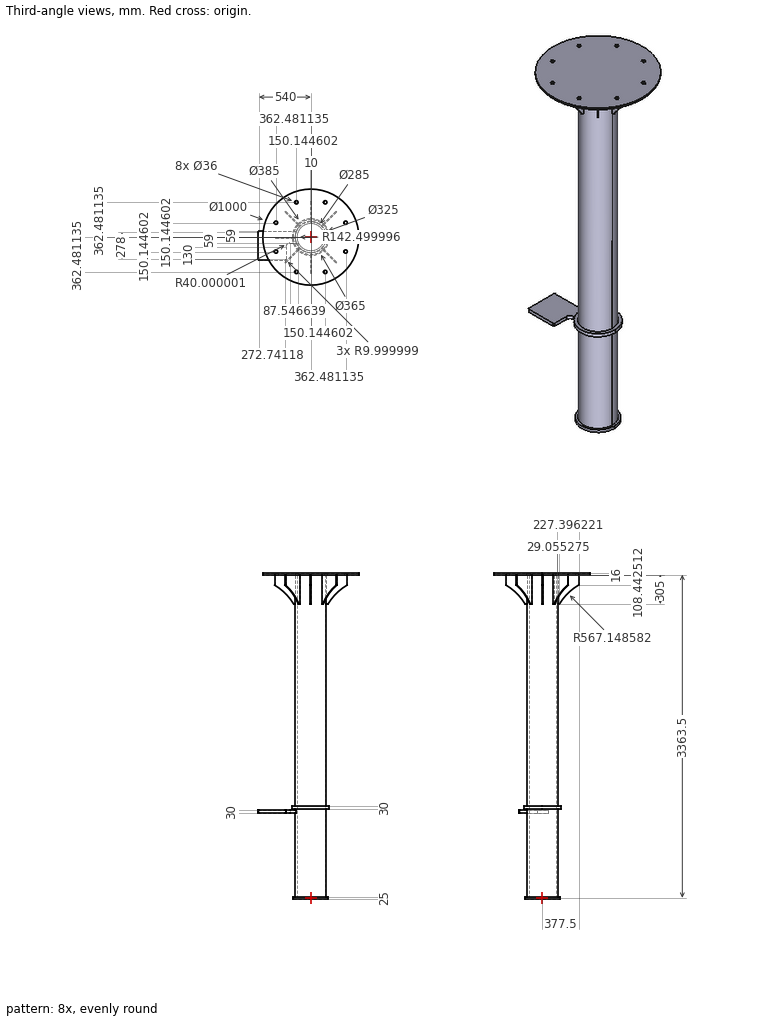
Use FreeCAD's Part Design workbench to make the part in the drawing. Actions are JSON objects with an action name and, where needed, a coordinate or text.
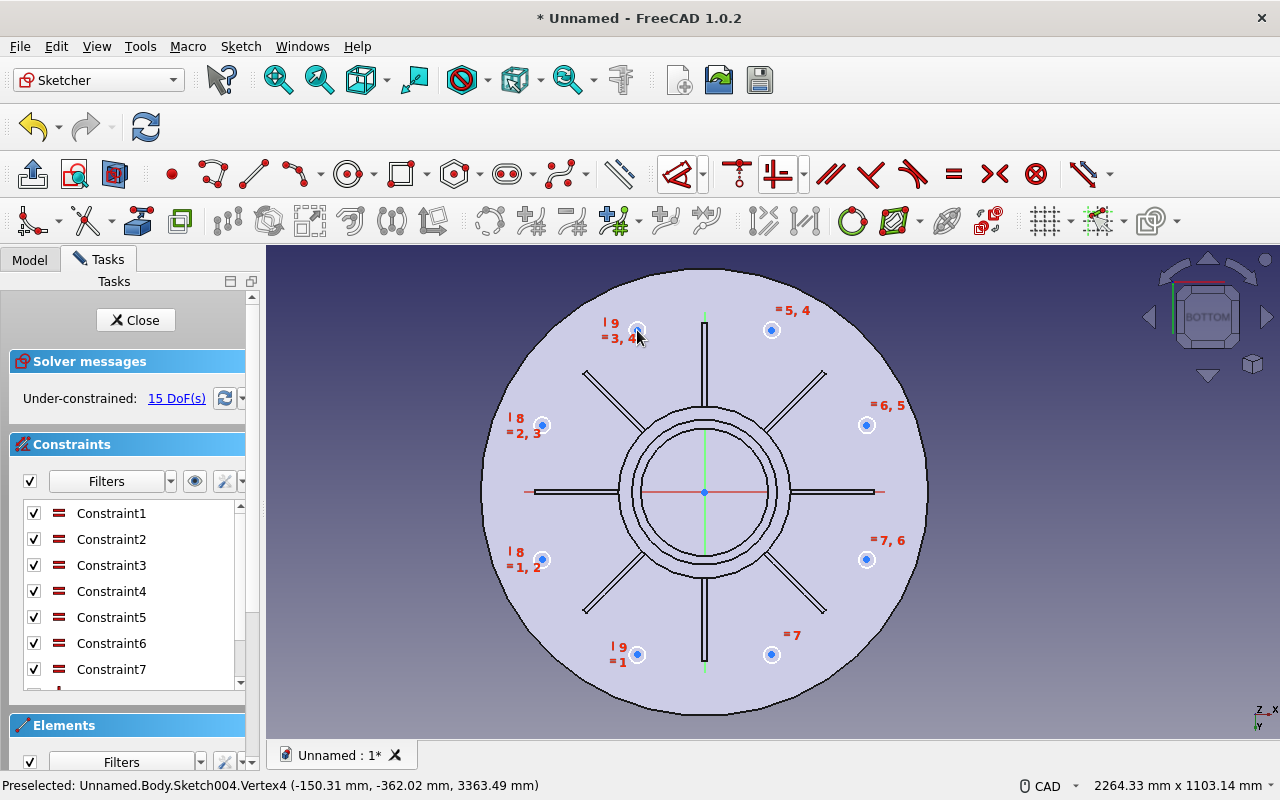
{"action": "left_click", "coordinate": [637, 330]}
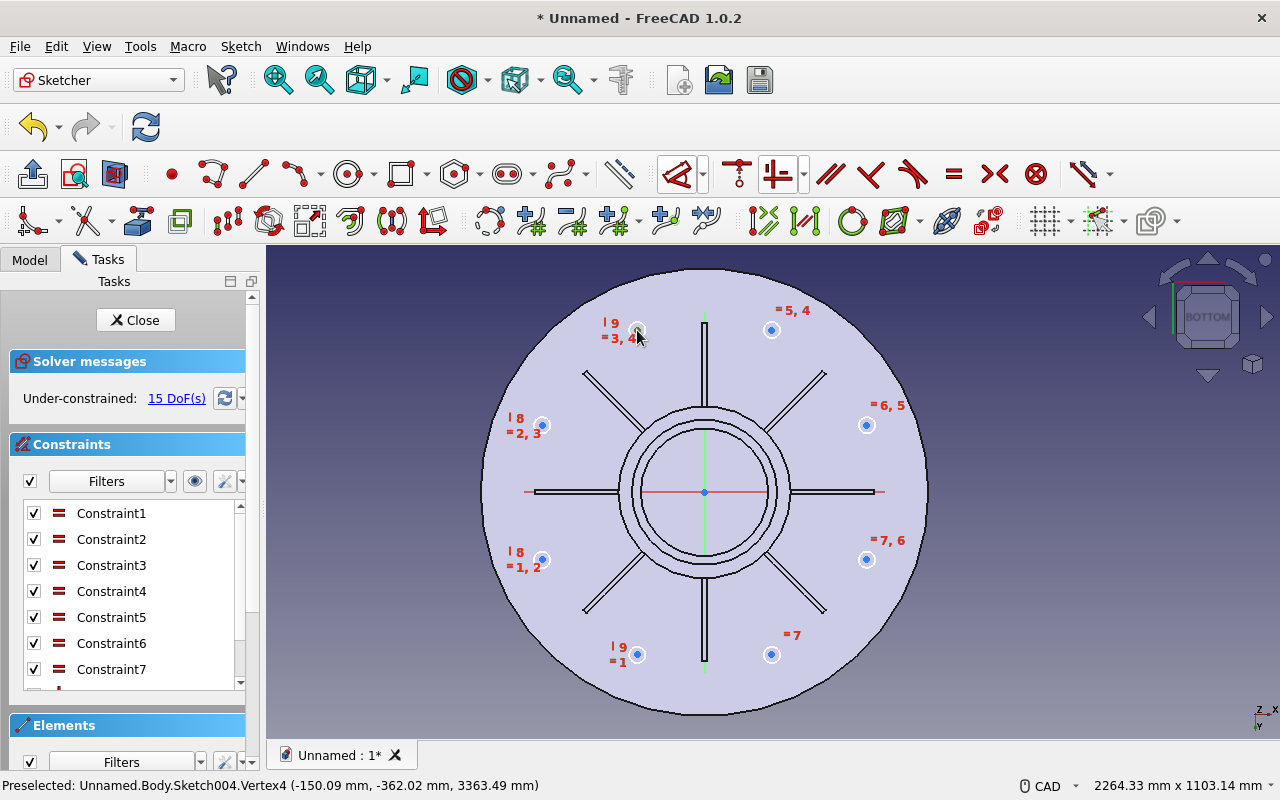
{"action": "left_click", "coordinate": [772, 330]}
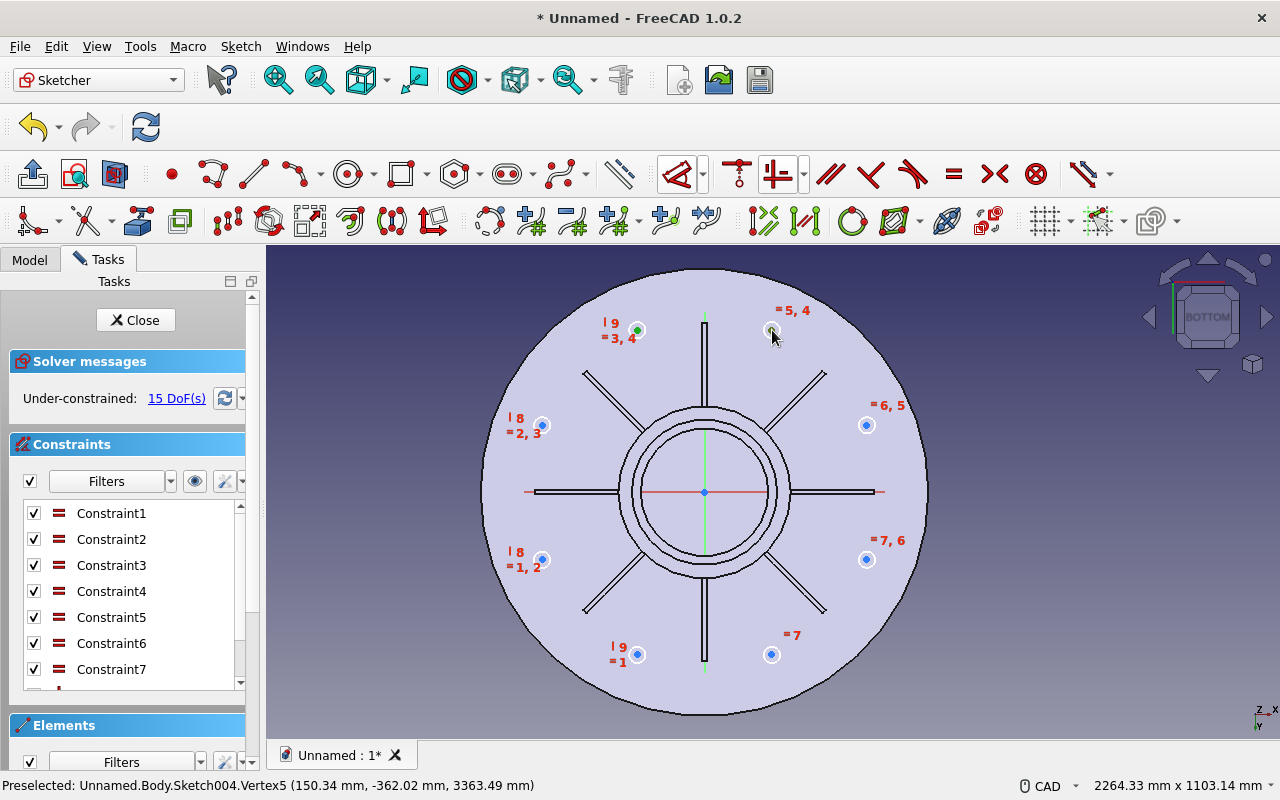
{"action": "key", "text": "h"}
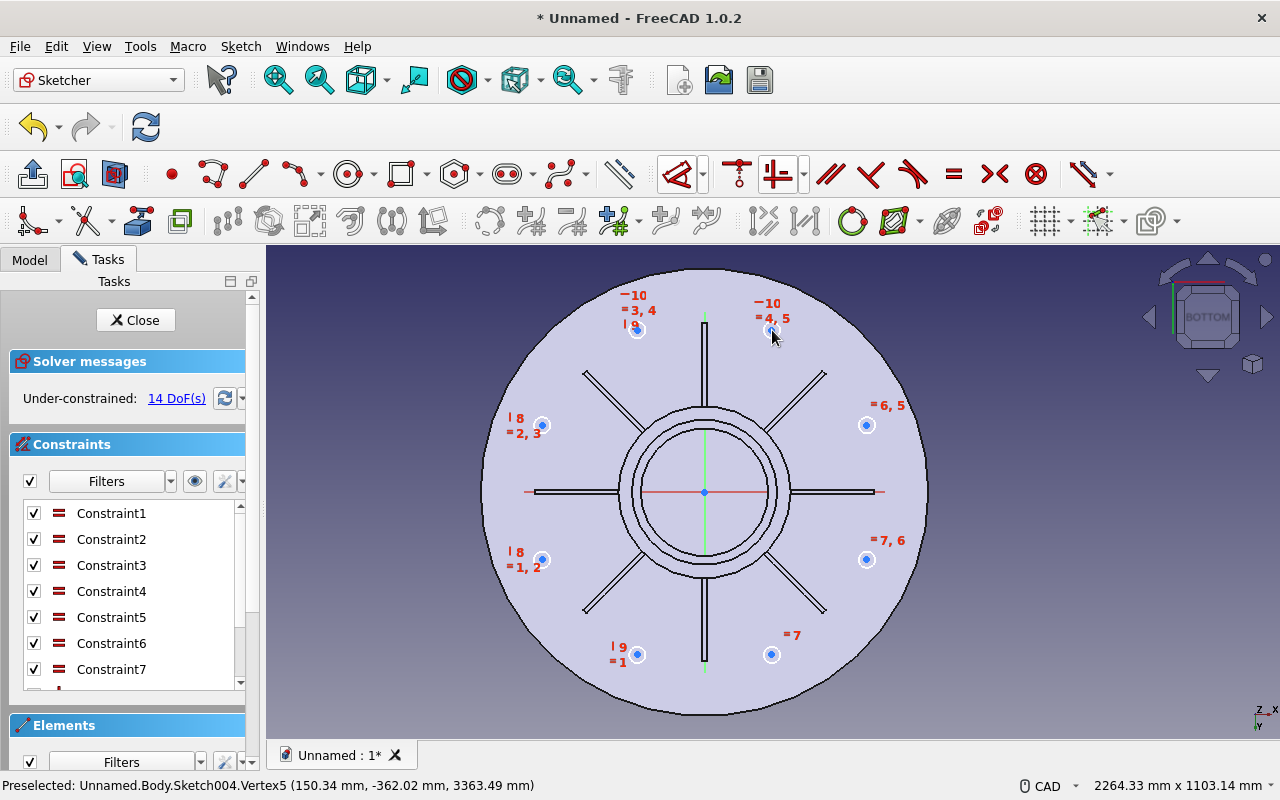
{"action": "left_click", "coordinate": [542, 425]}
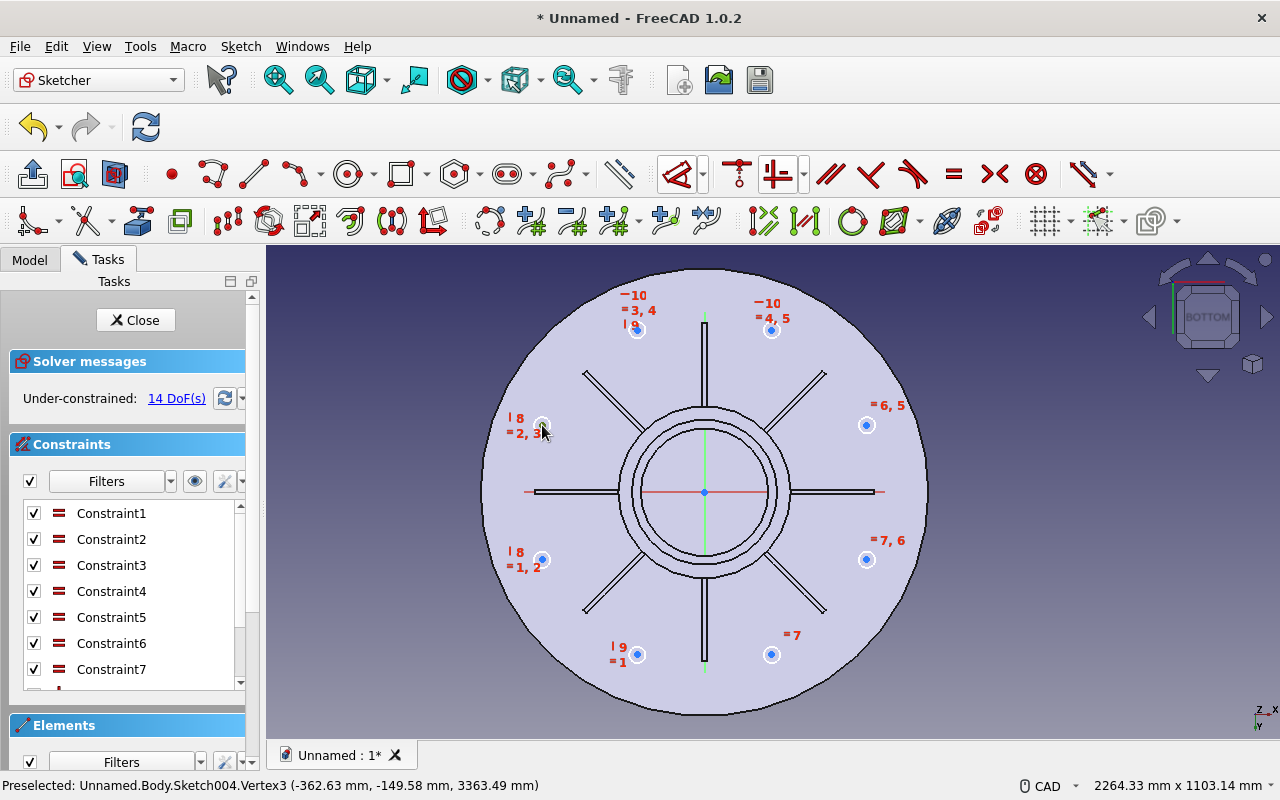
{"action": "left_click", "coordinate": [867, 425]}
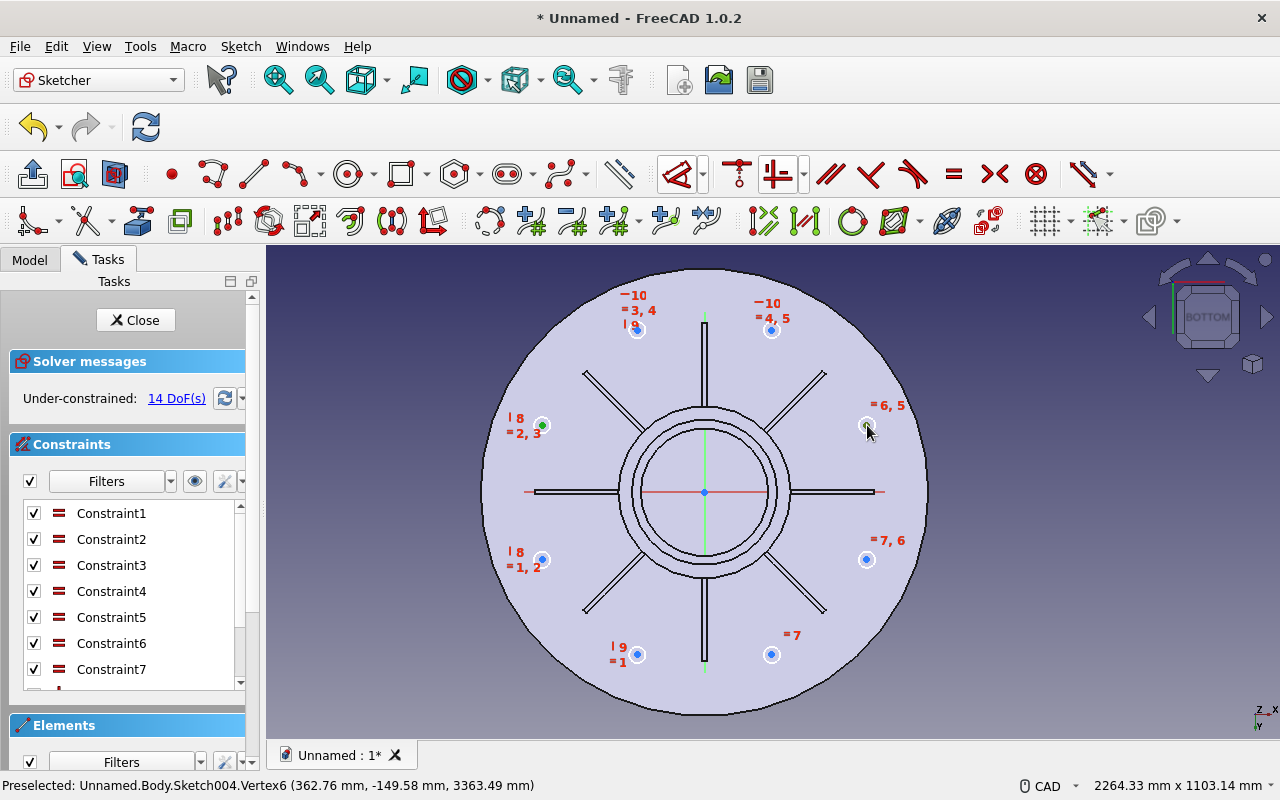
{"action": "key", "text": "h"}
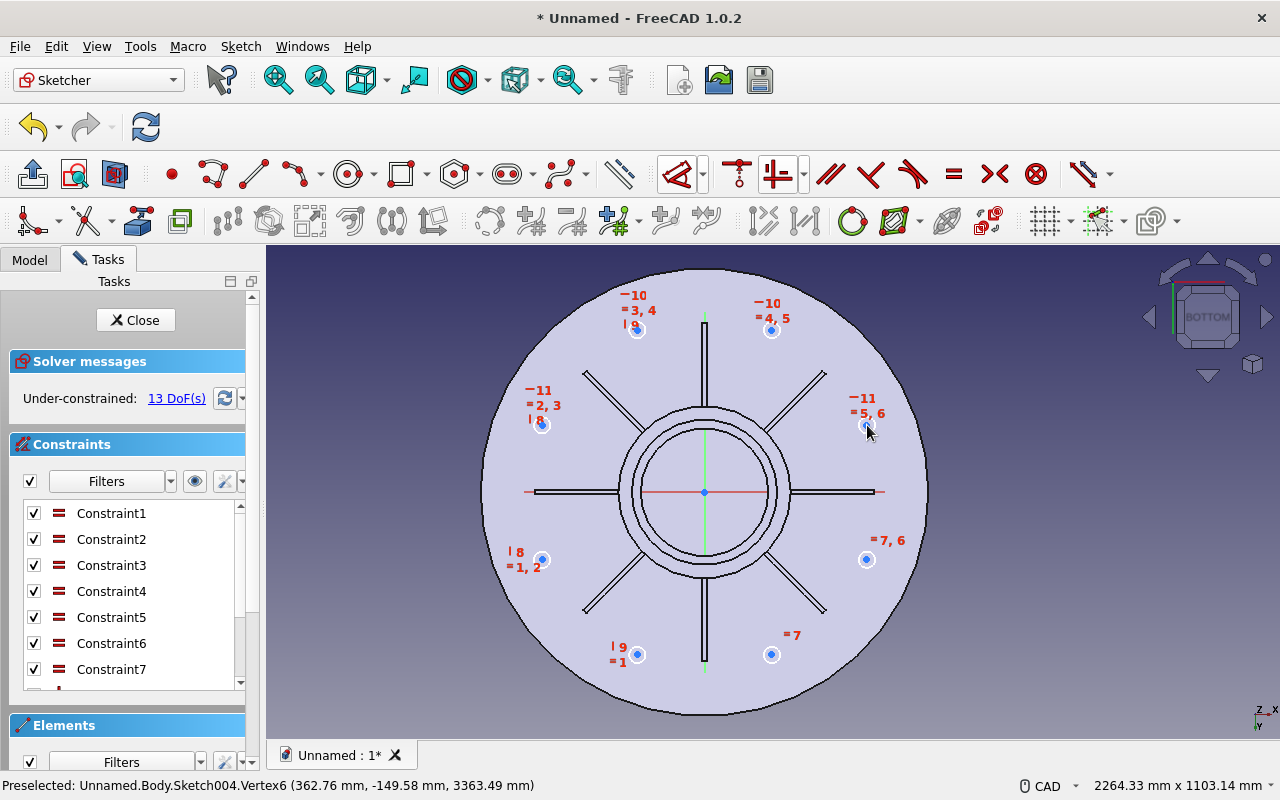
{"action": "left_click", "coordinate": [867, 425]}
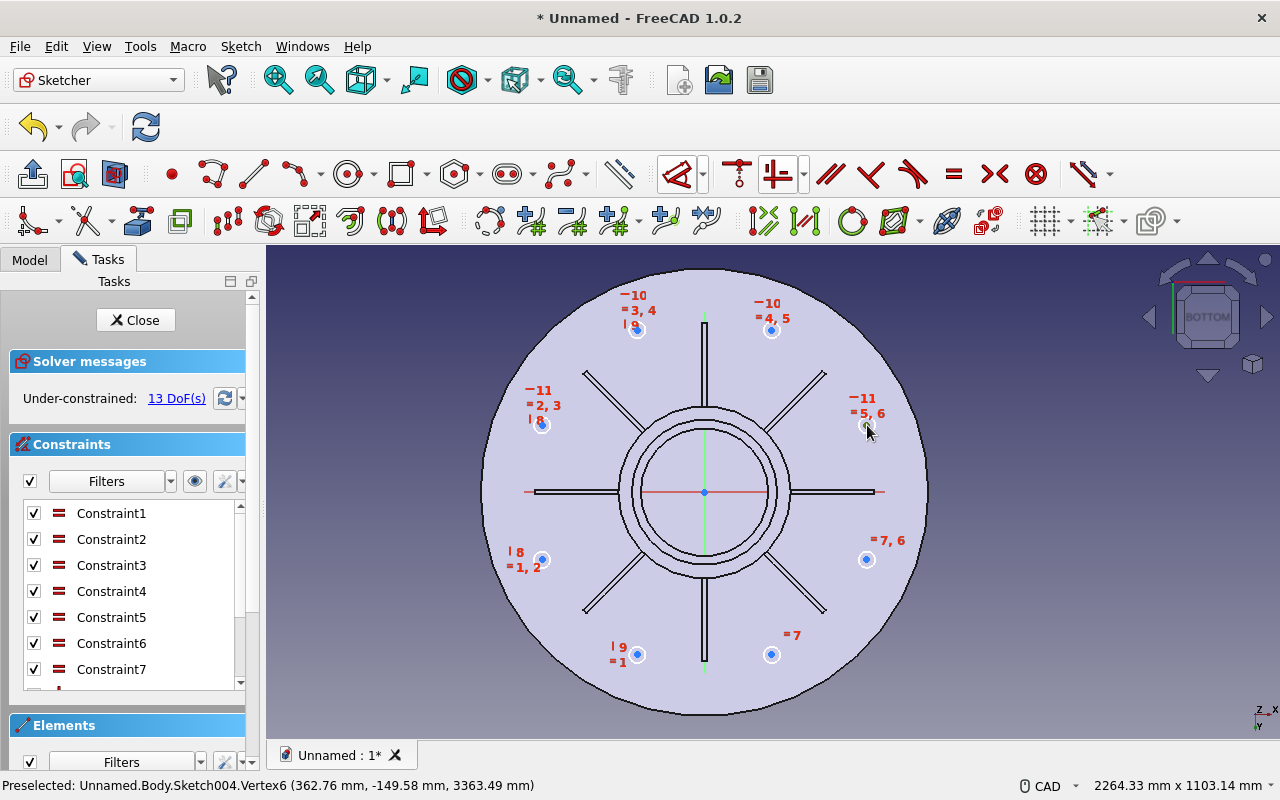
{"action": "left_click", "coordinate": [867, 560]}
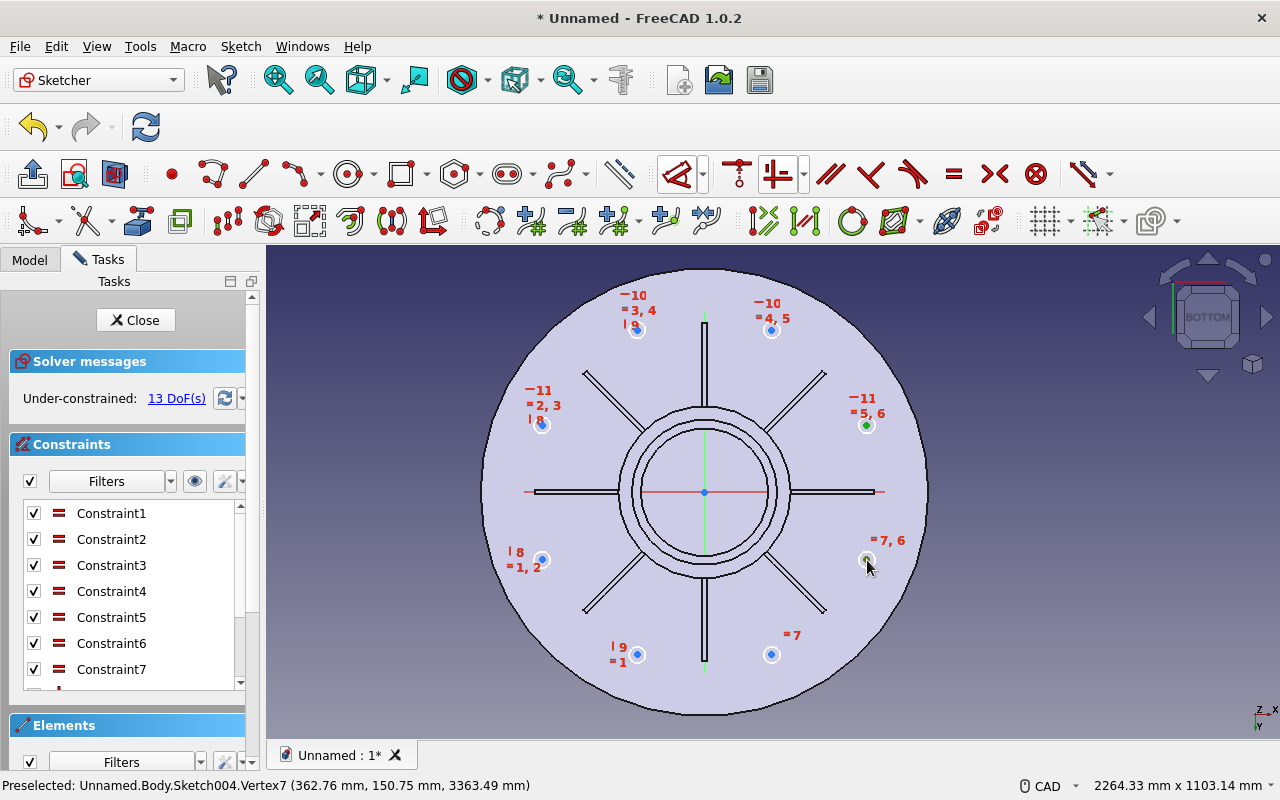
{"action": "key", "text": "v"}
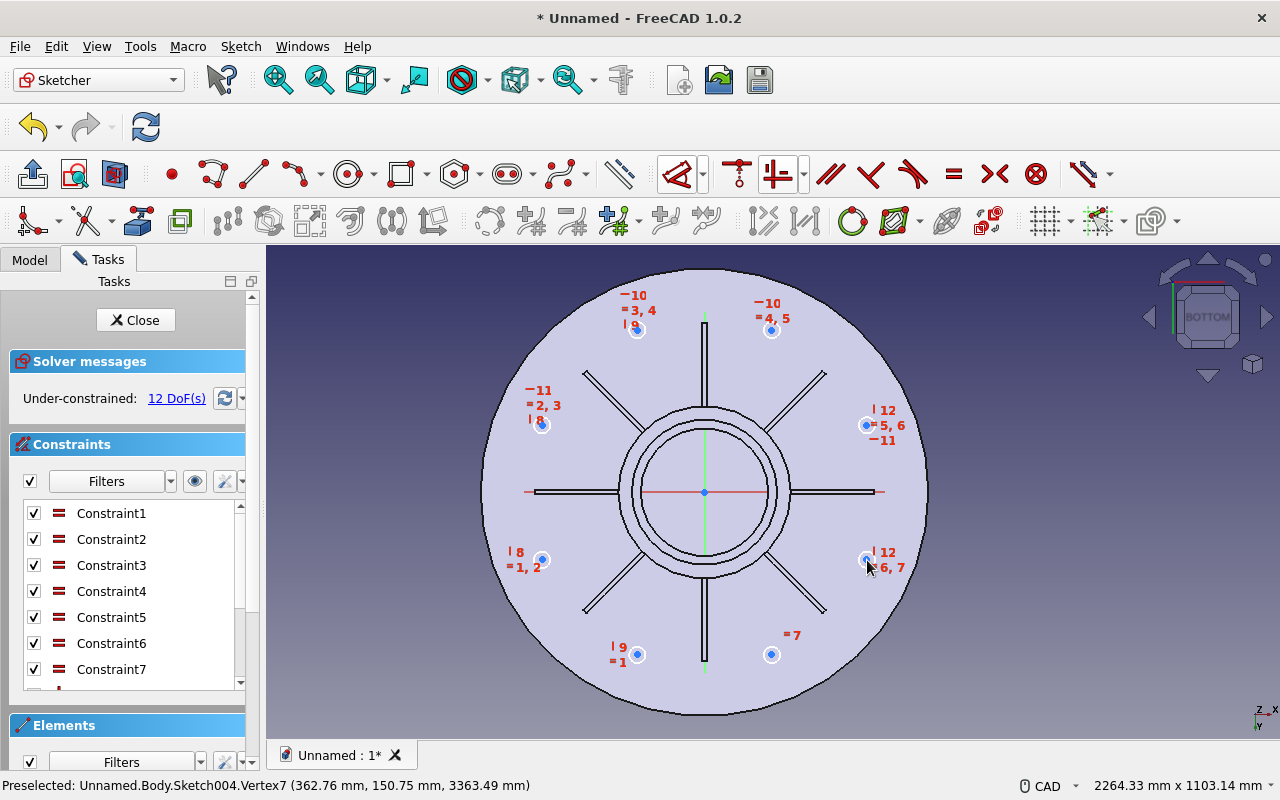
{"action": "left_click", "coordinate": [542, 560]}